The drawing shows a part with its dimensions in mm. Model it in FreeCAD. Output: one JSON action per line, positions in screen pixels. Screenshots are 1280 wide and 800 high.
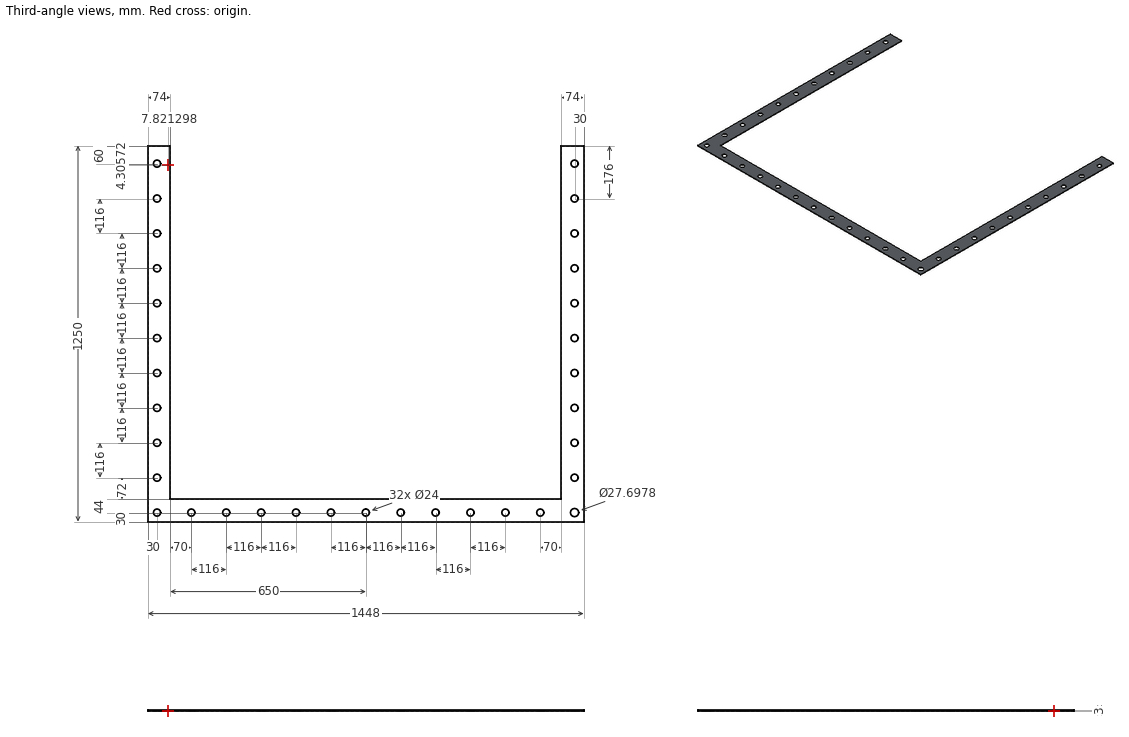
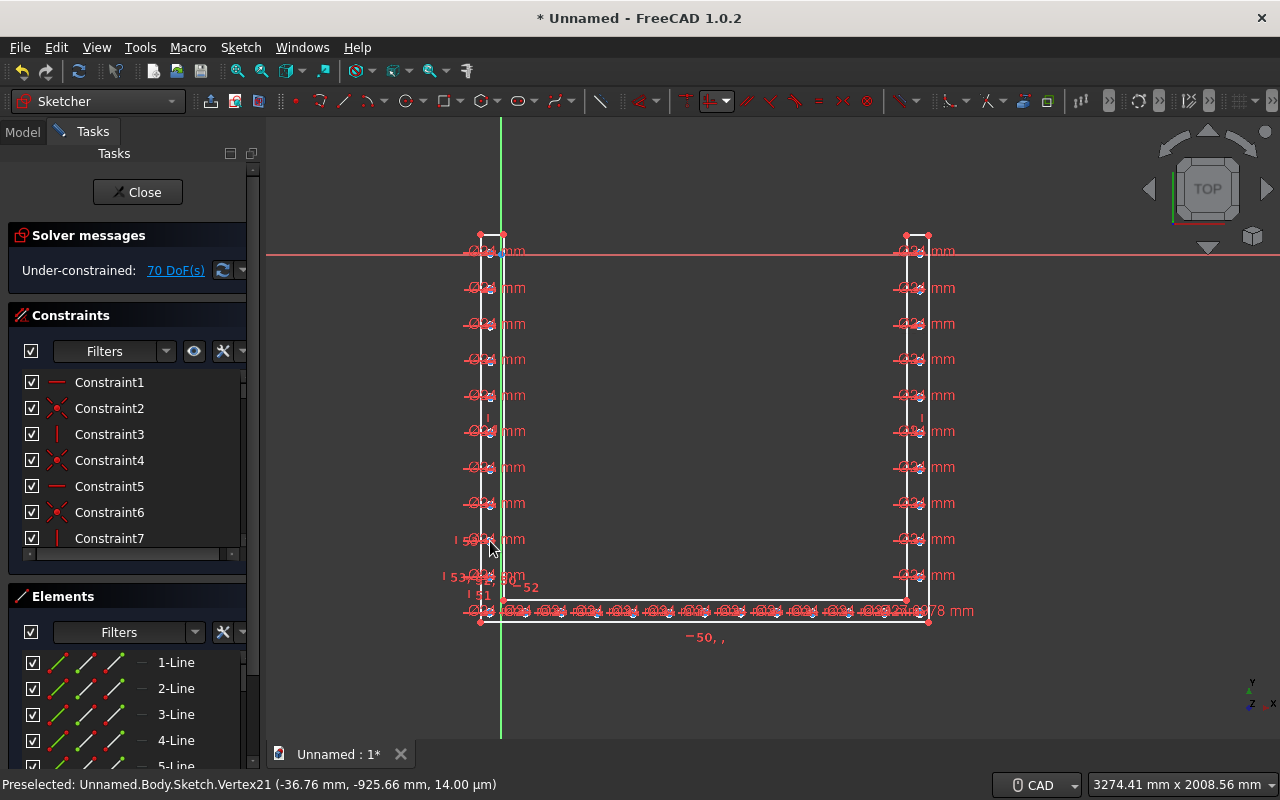
{"action": "left_click", "coordinate": [526, 613]}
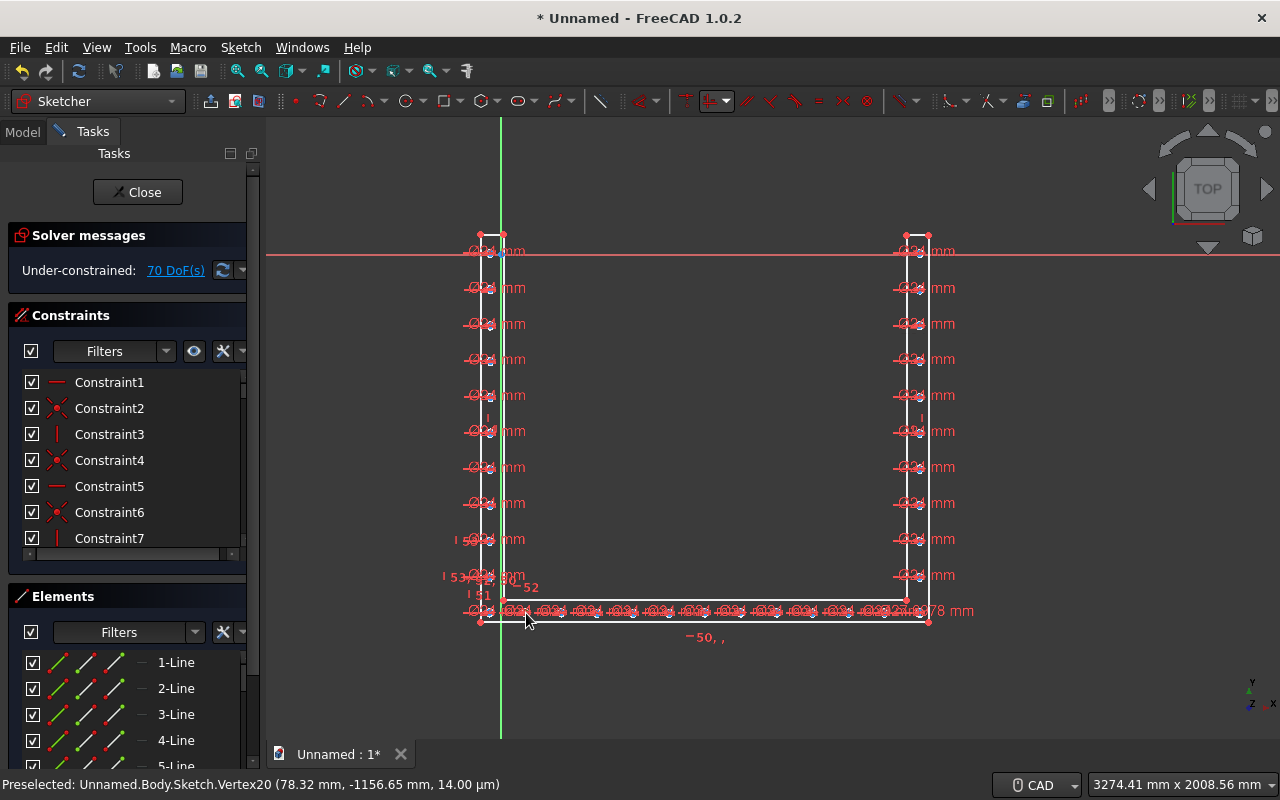
{"action": "left_click", "coordinate": [561, 613]}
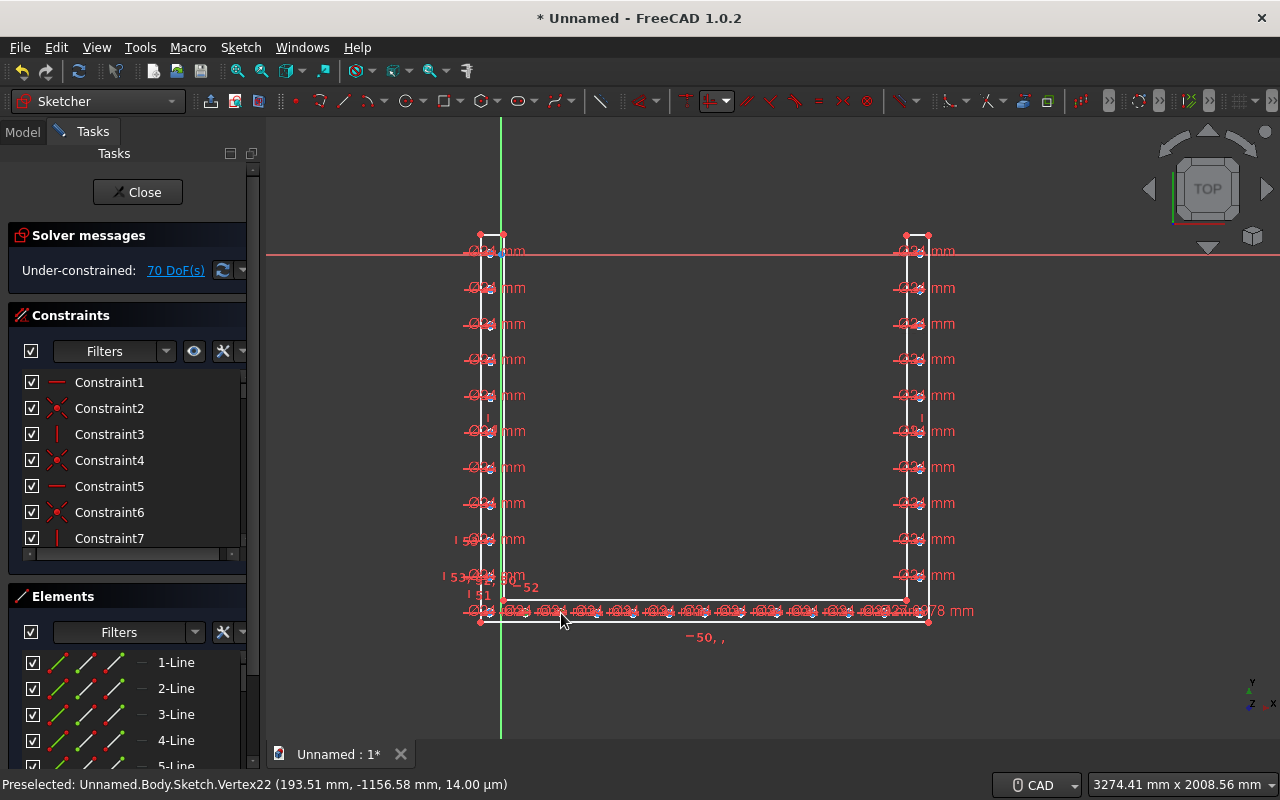
{"action": "key", "text": "h"}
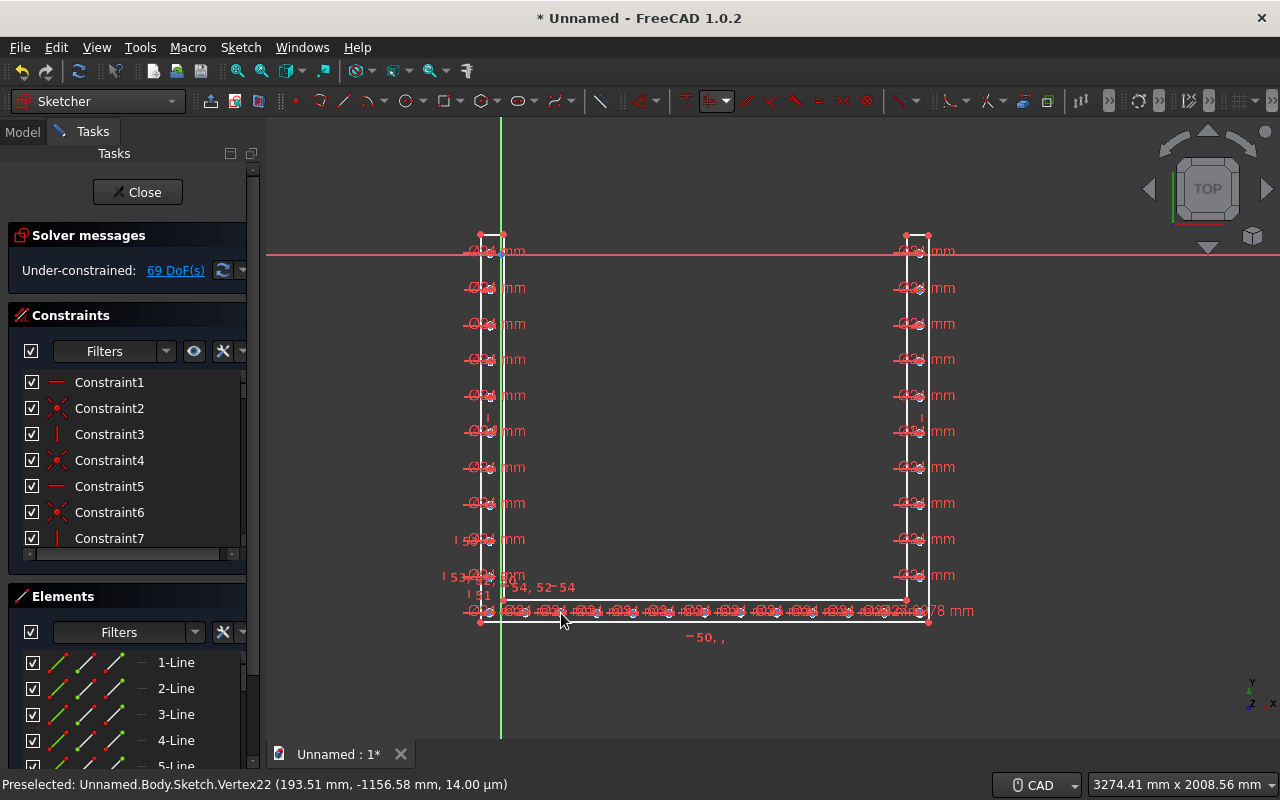
{"action": "left_click", "coordinate": [490, 541]}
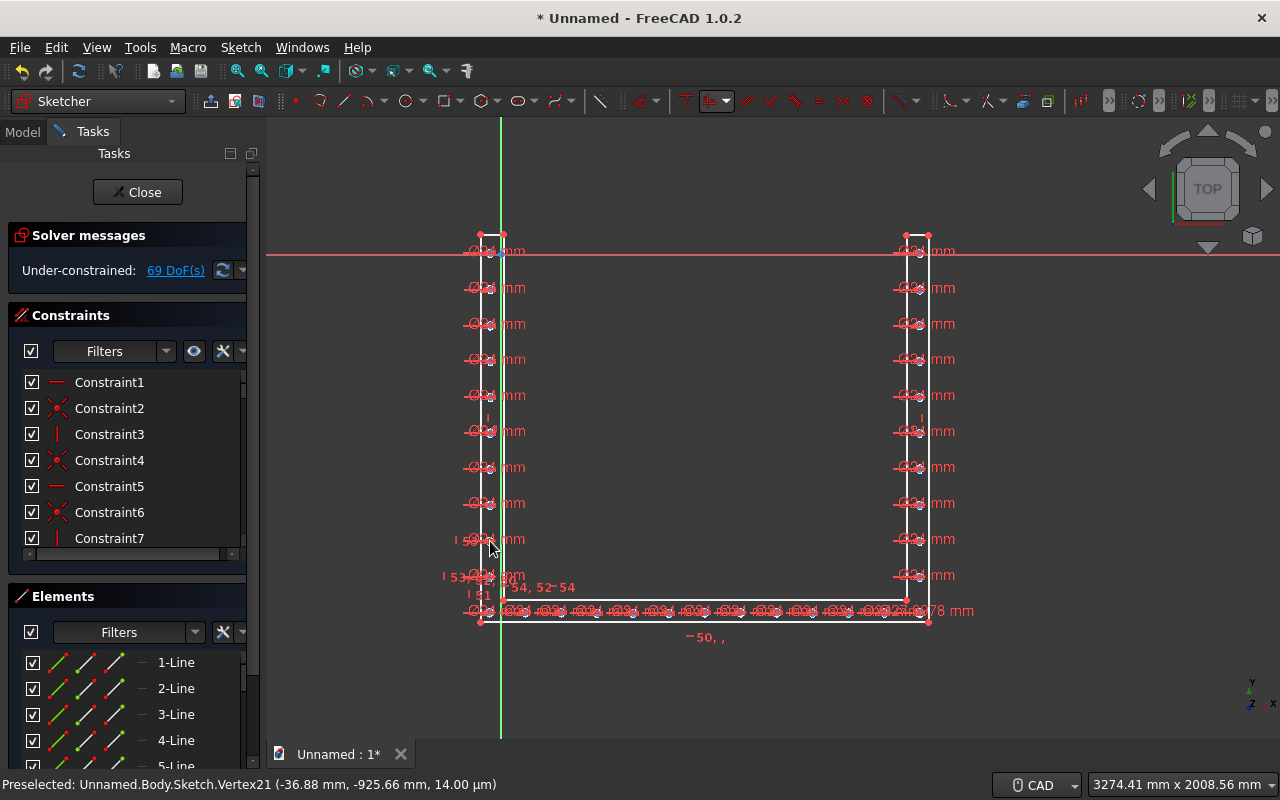
{"action": "left_click", "coordinate": [490, 505]}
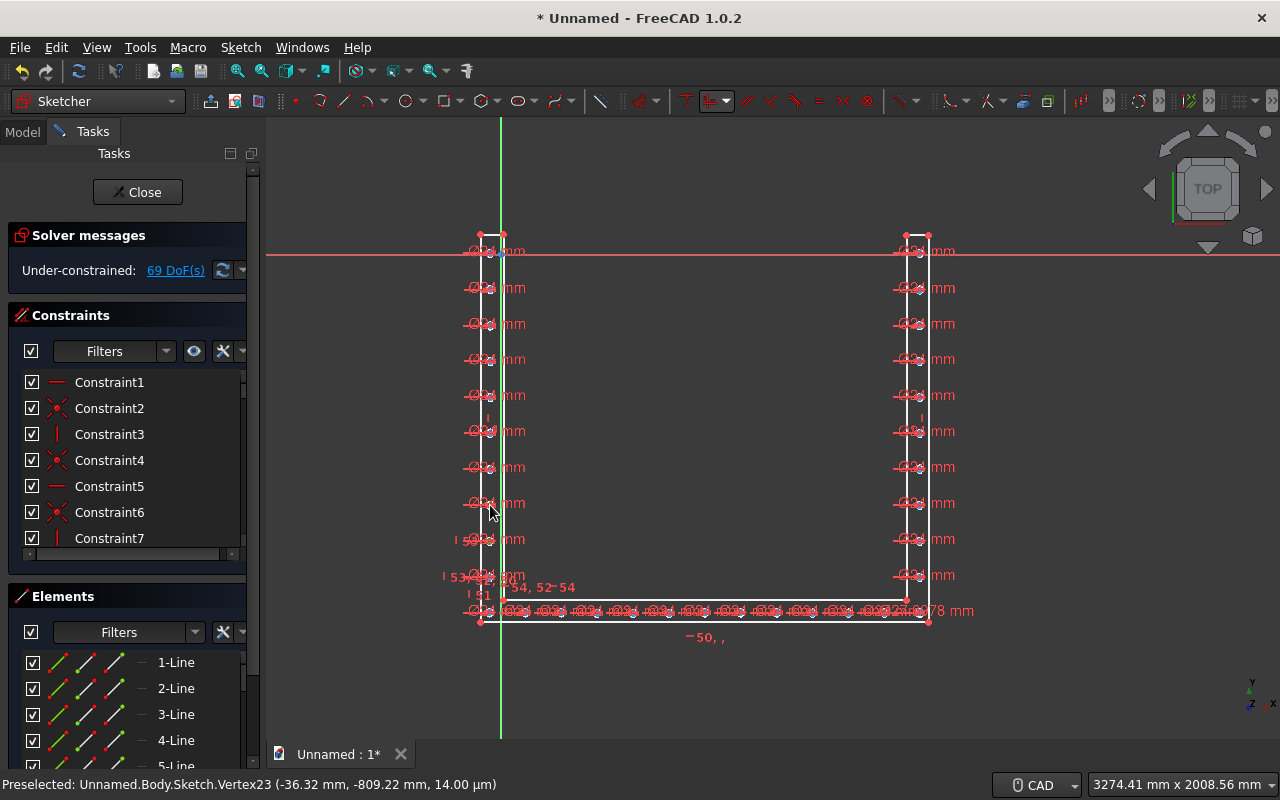
{"action": "left_click", "coordinate": [728, 102]}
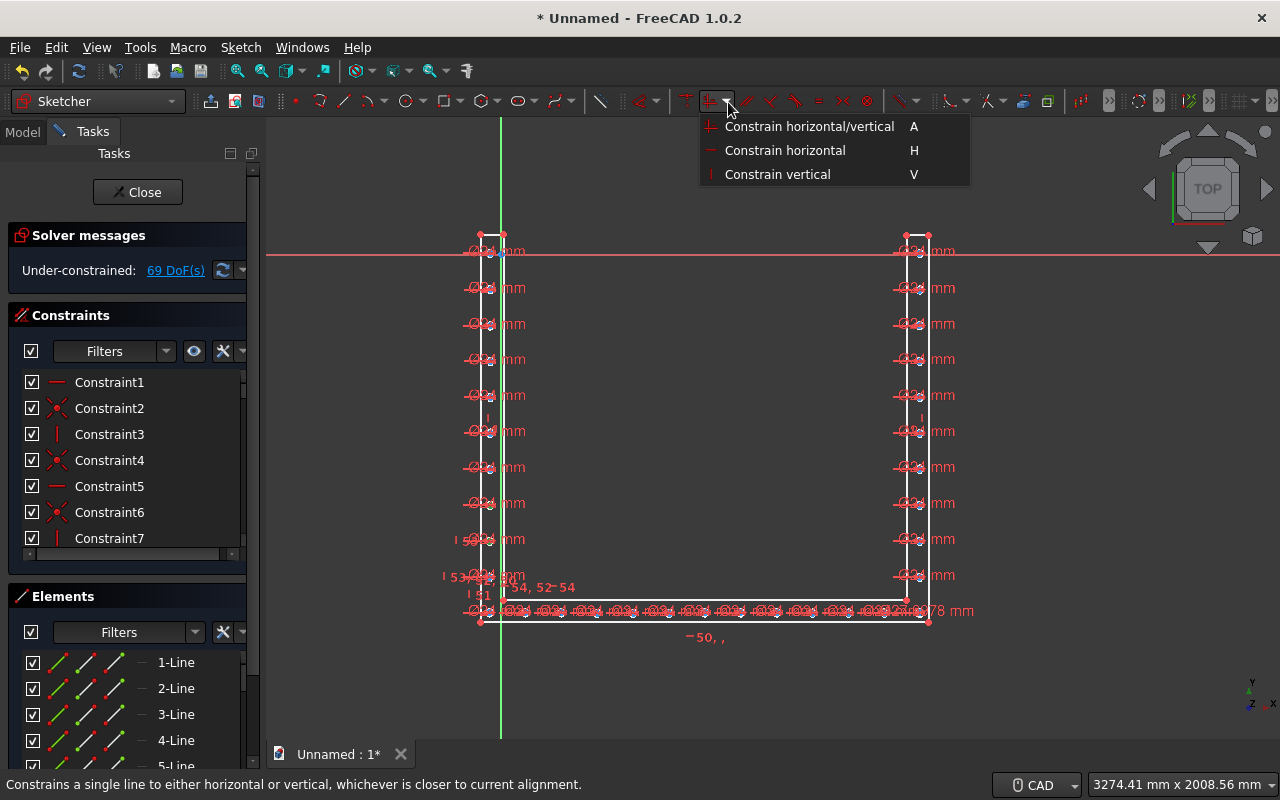
{"action": "left_click", "coordinate": [835, 174]}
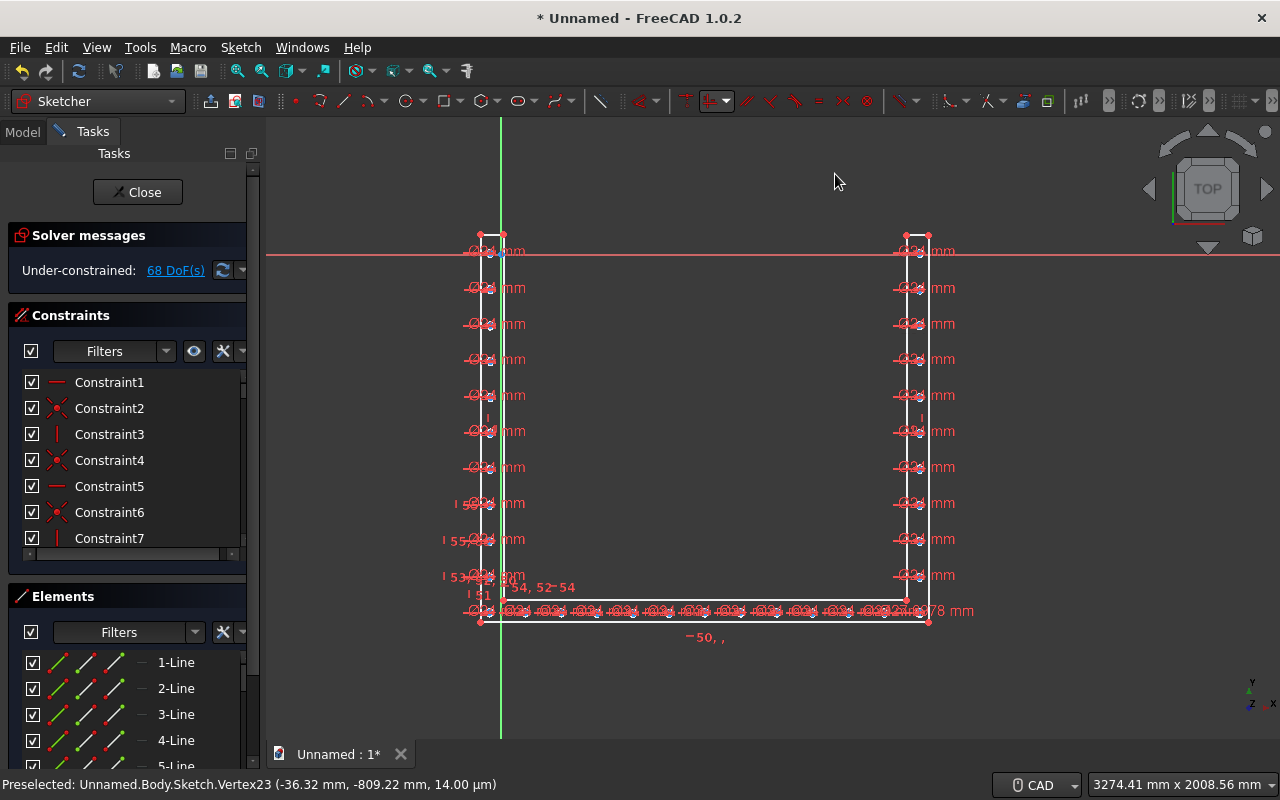
{"action": "left_click", "coordinate": [490, 505]}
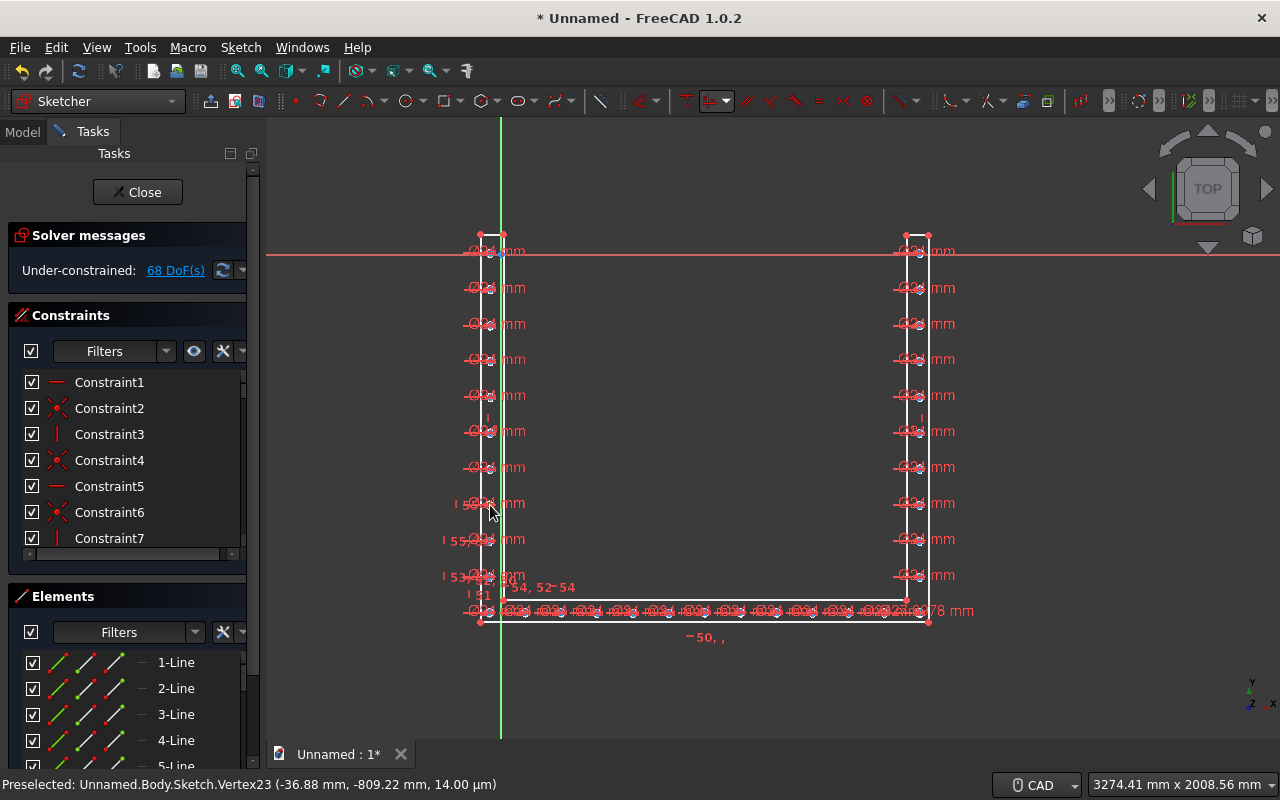
{"action": "left_click", "coordinate": [490, 469]}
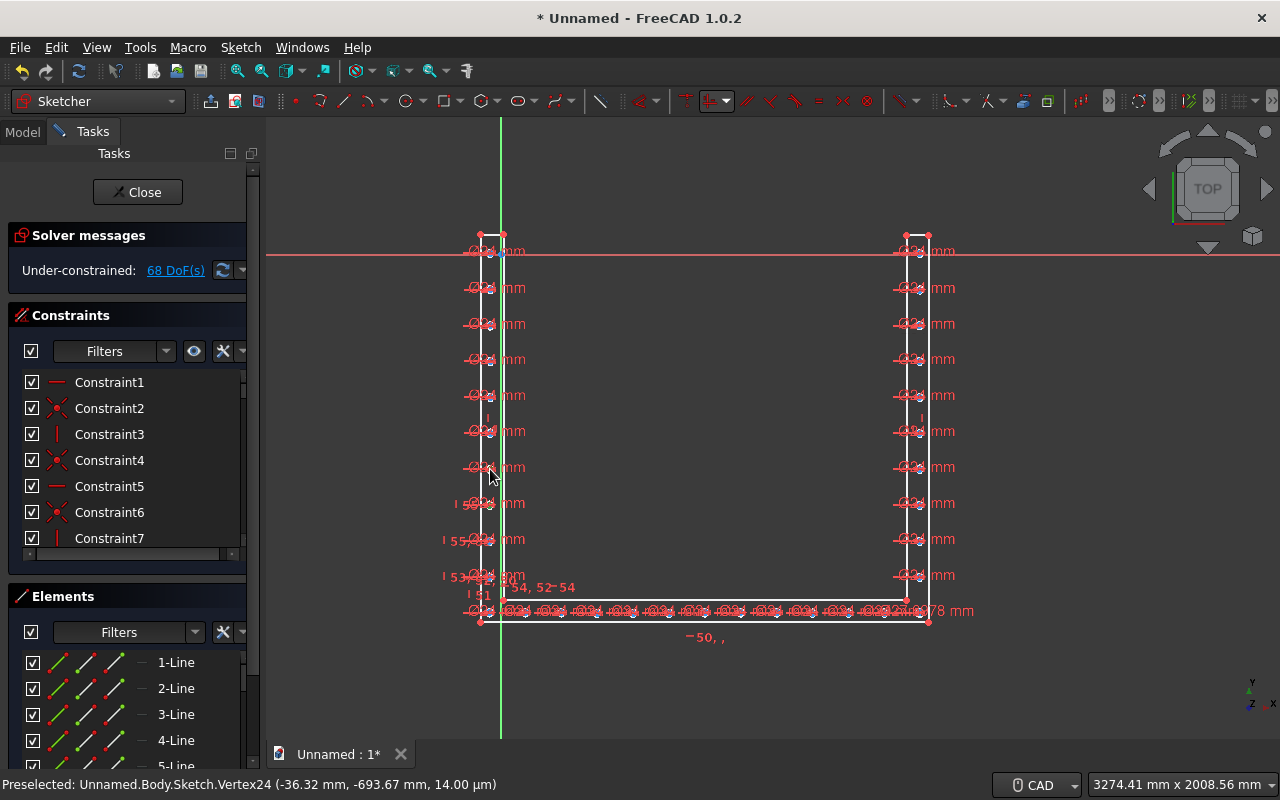
{"action": "left_click", "coordinate": [728, 102]}